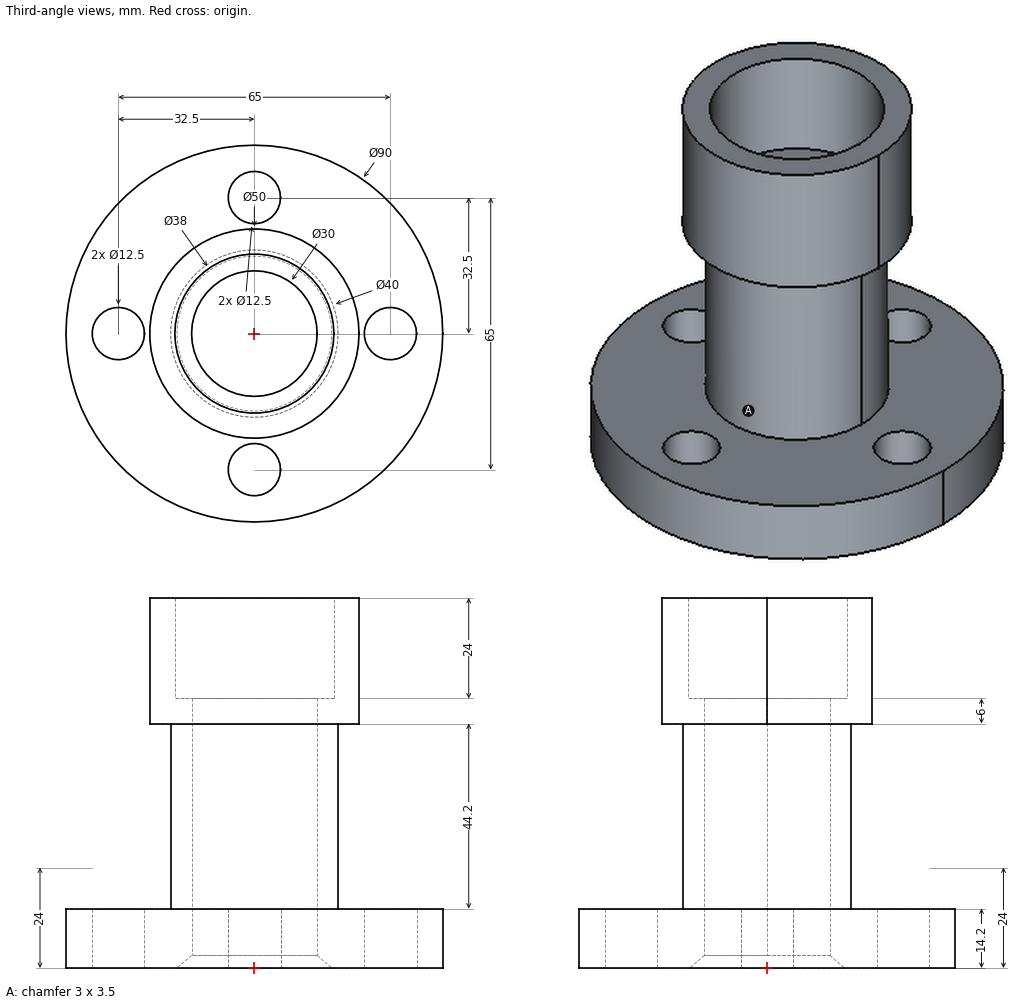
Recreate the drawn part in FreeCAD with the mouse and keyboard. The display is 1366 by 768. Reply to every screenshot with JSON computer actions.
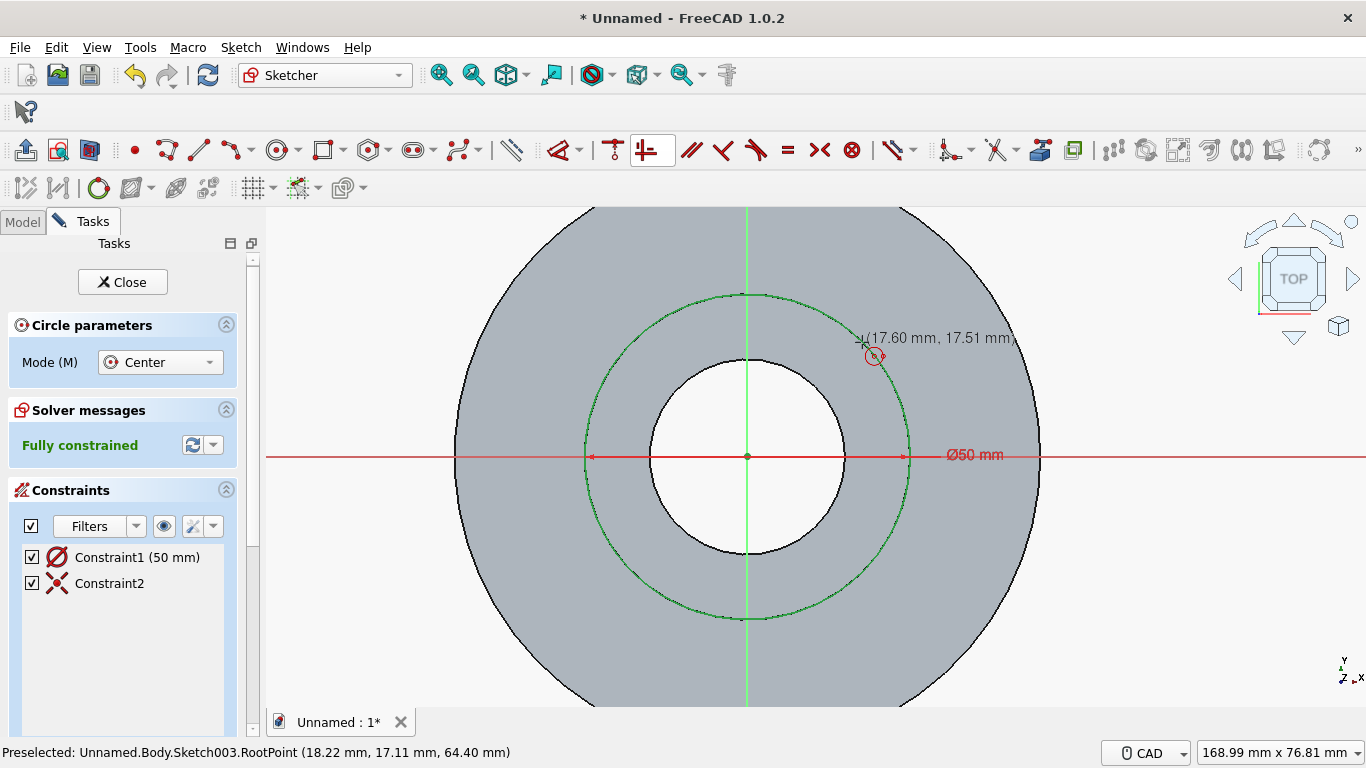
{"action": "left_click", "coordinate": [747, 457]}
{"action": "mouse_move", "coordinate": [835, 370]}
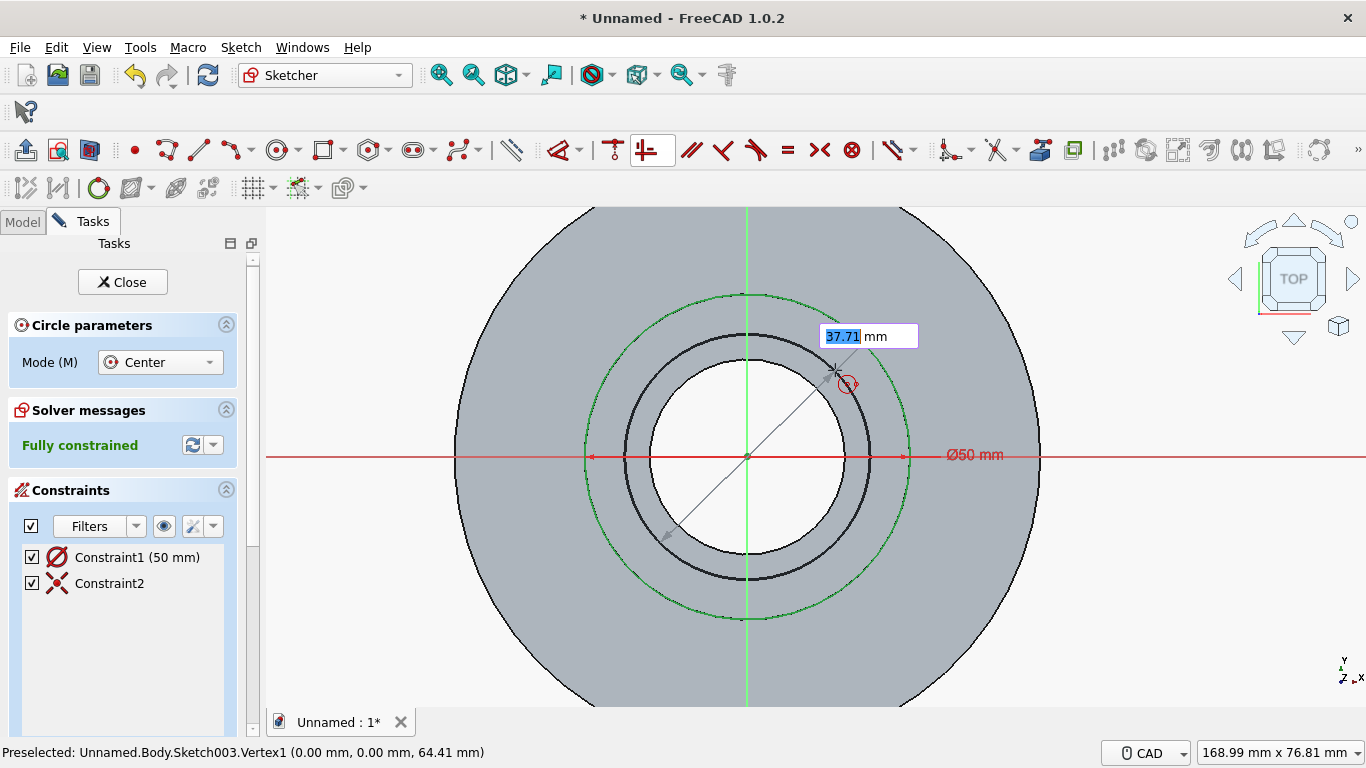
{"action": "type", "text": "38"}
{"action": "key", "text": "Return"}
{"action": "key", "text": "Escape"}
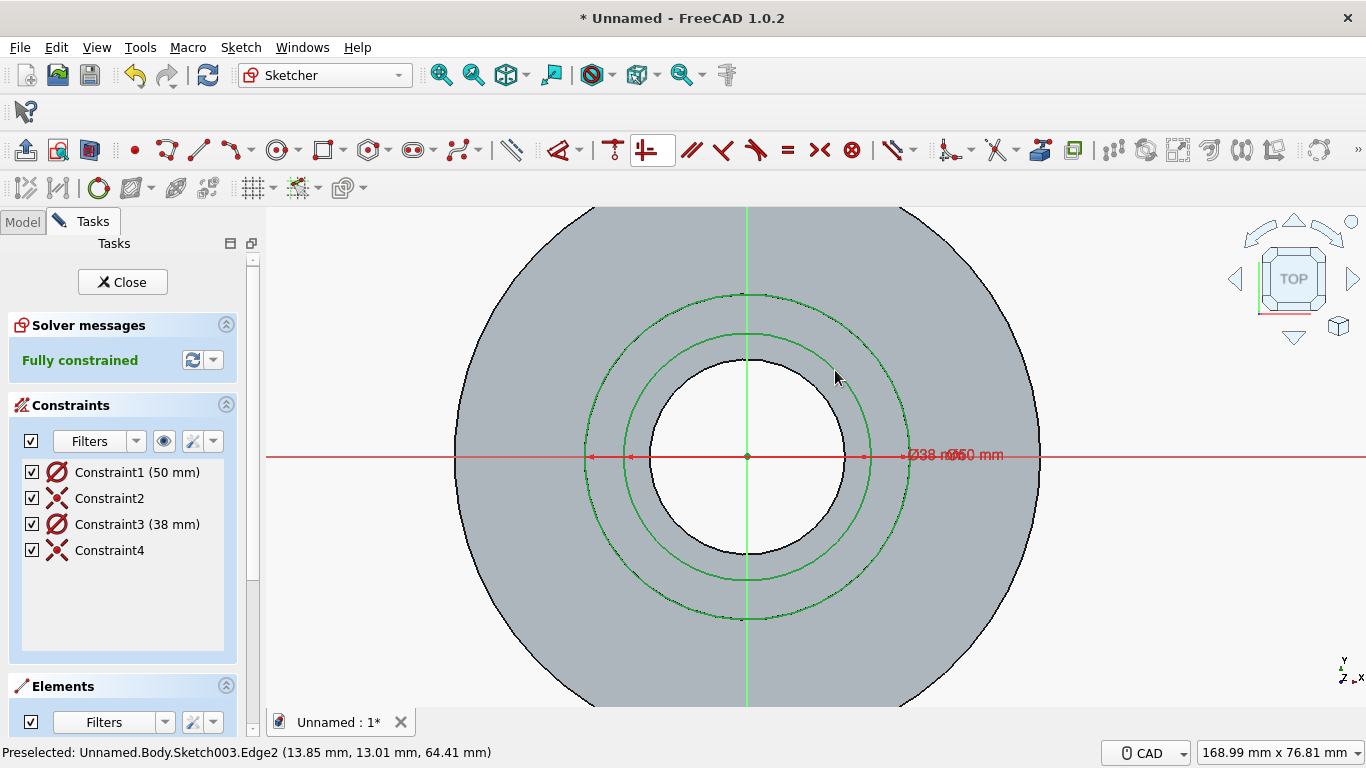
{"action": "left_click", "coordinate": [123, 282]}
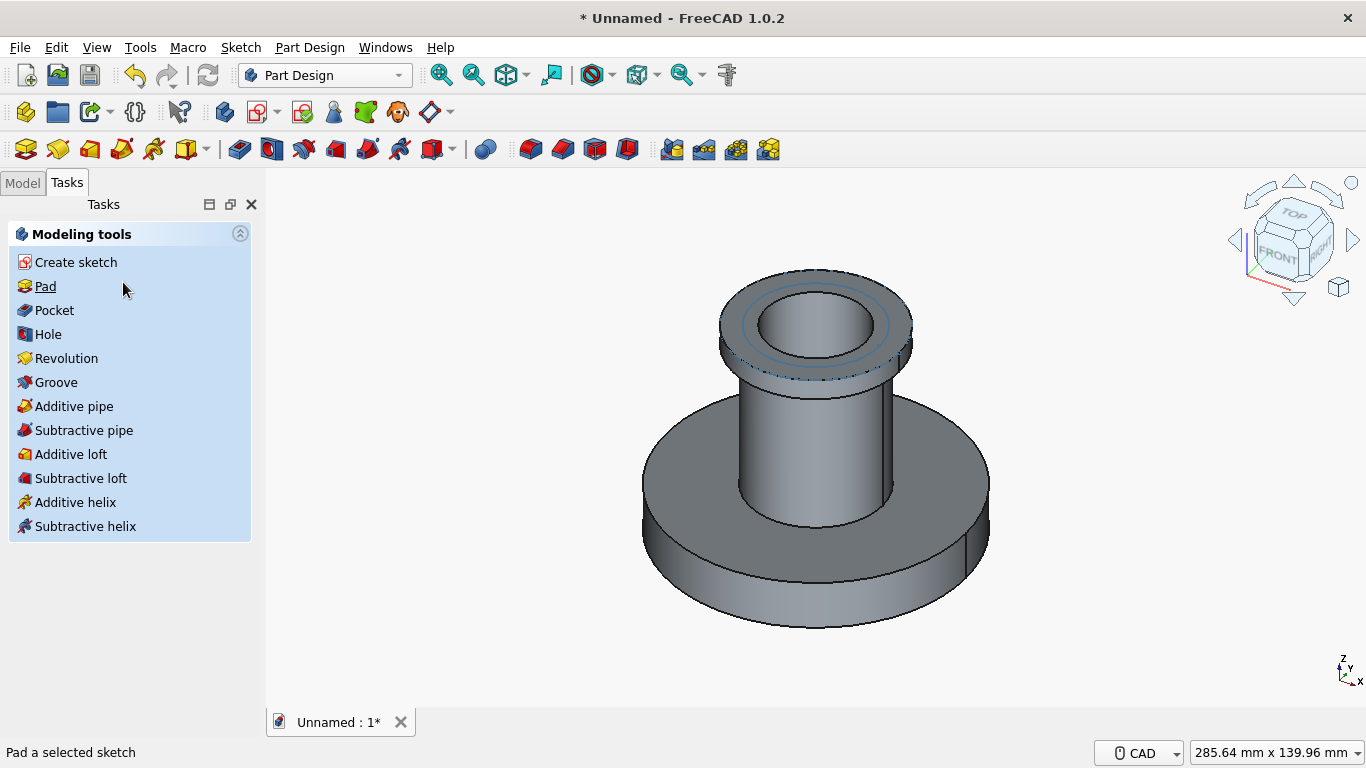
{"action": "left_click", "coordinate": [26, 150]}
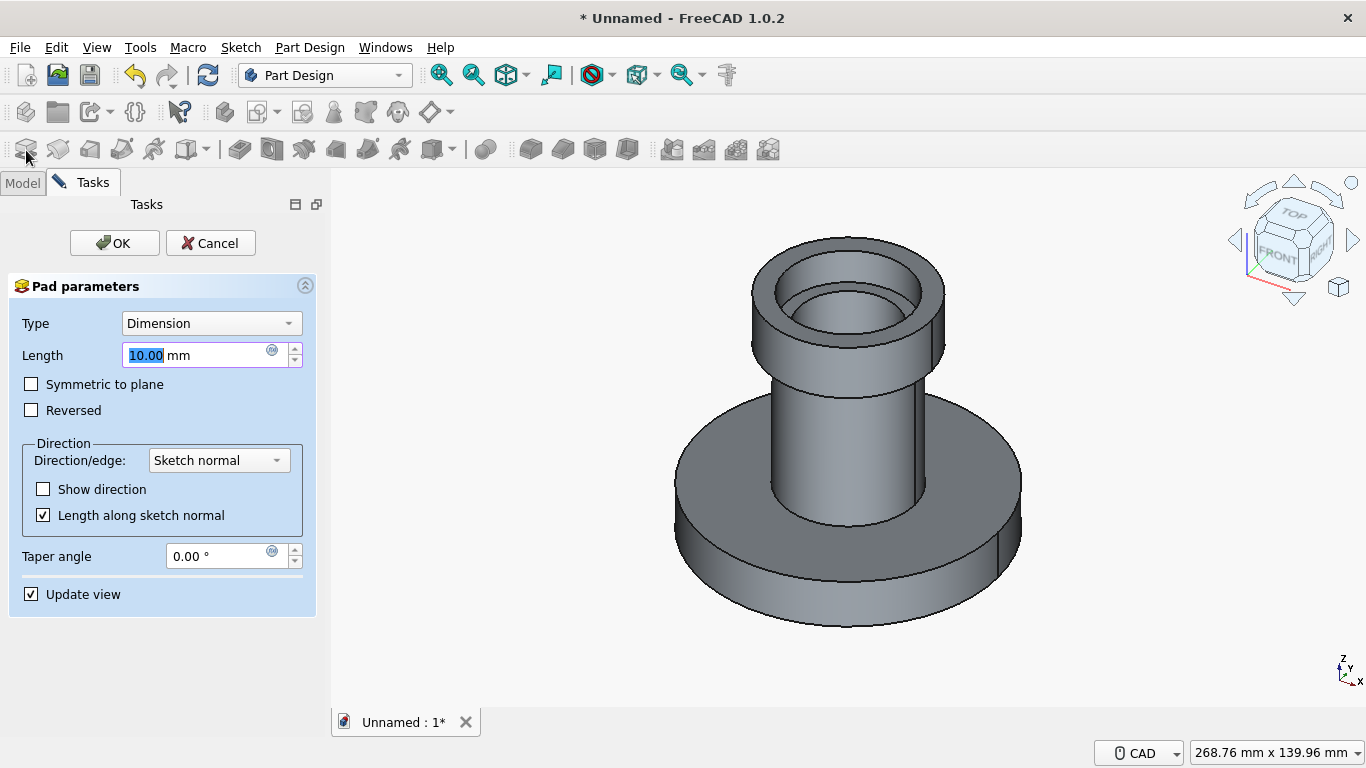
{"action": "type", "text": "24"}
{"action": "key", "text": "Tab"}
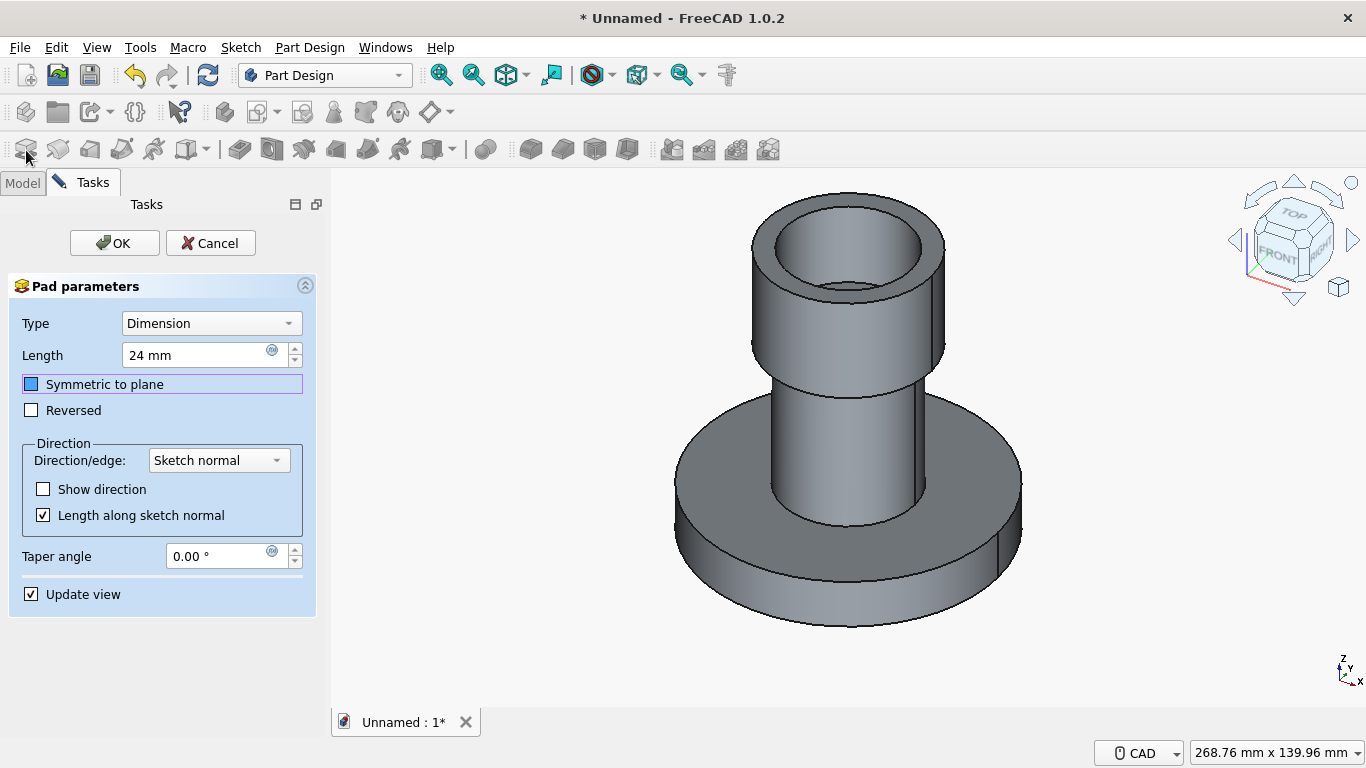
{"action": "left_click", "coordinate": [115, 243]}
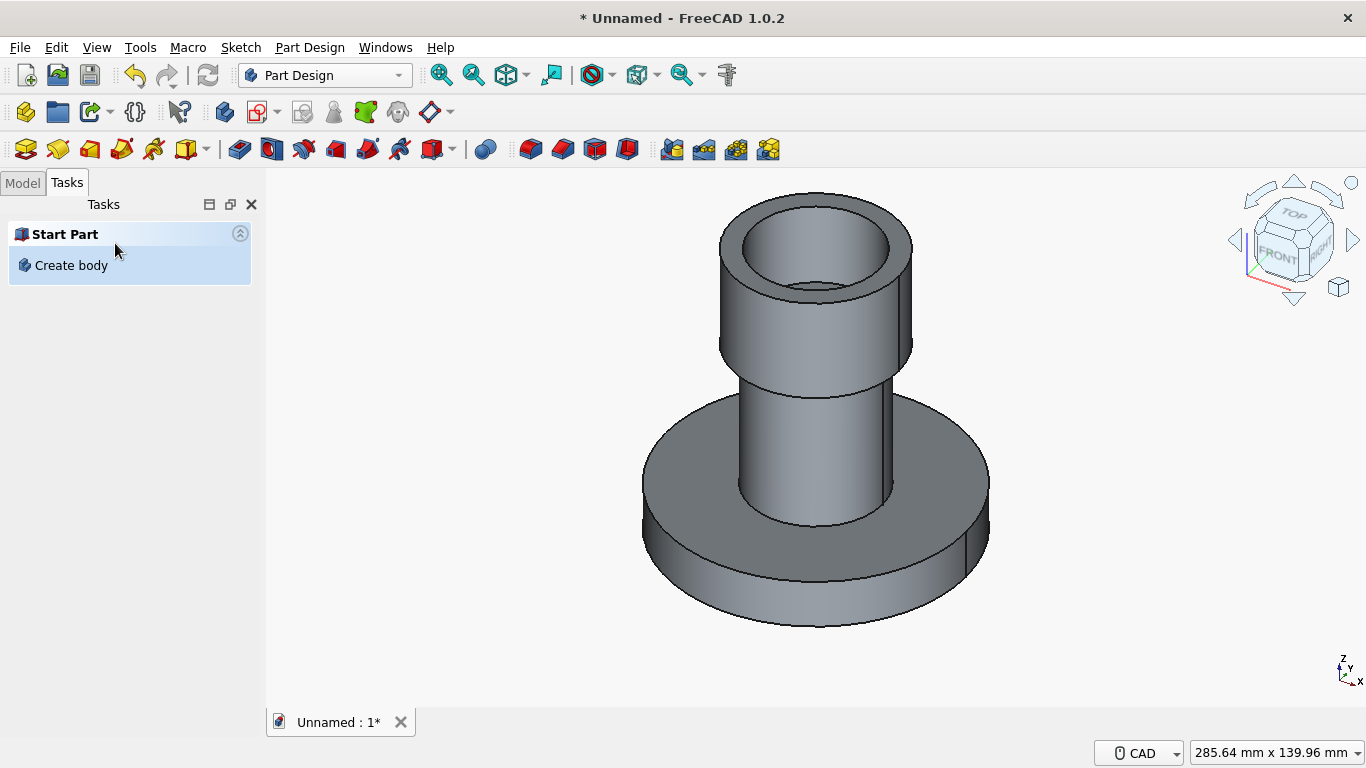
{"action": "key", "text": "v f"}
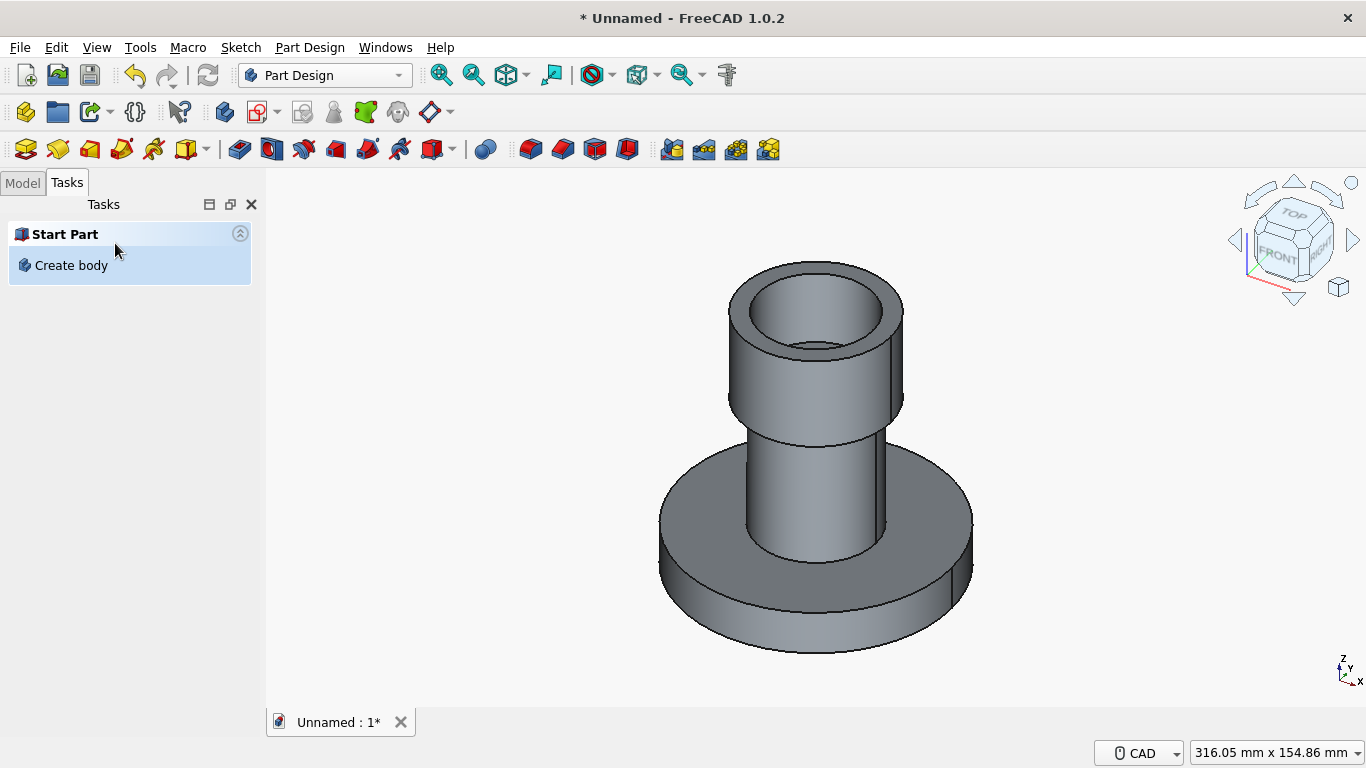
{"action": "key", "text": "0"}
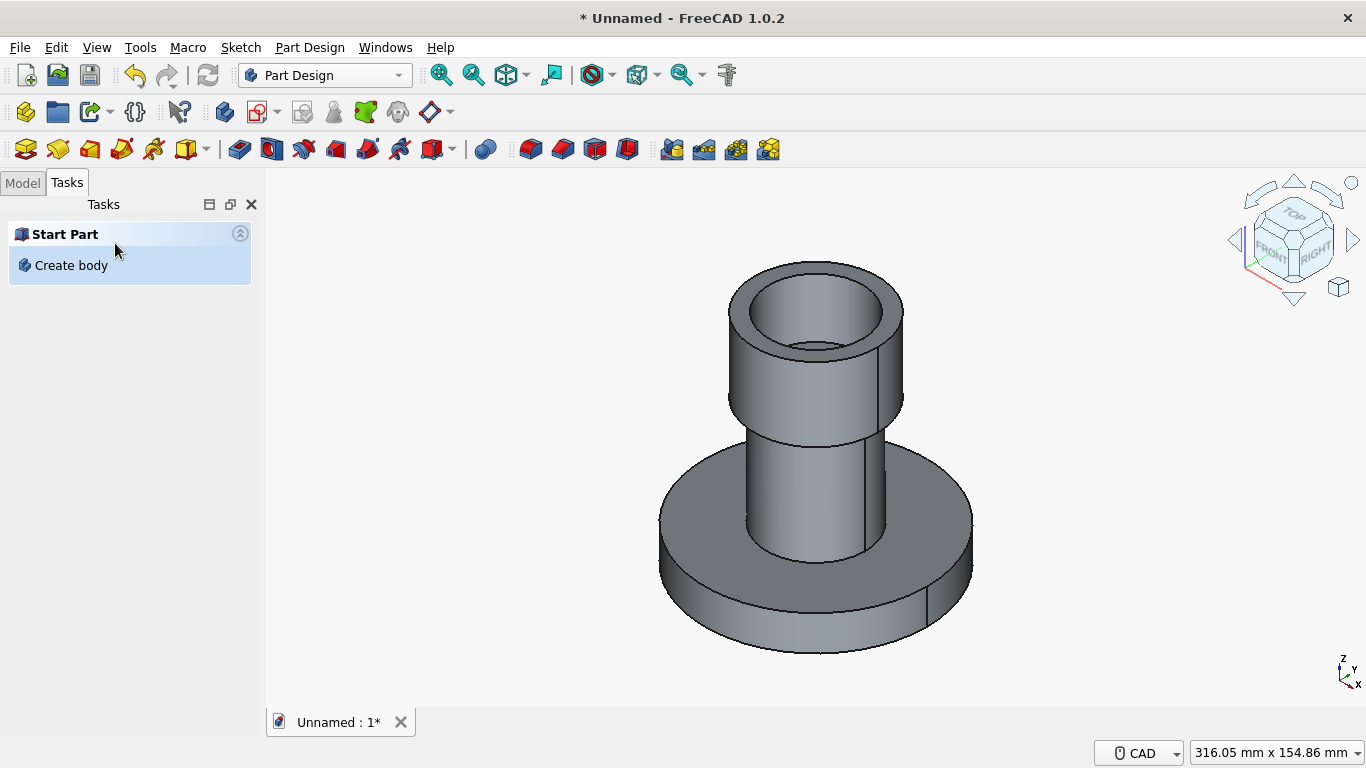
{"action": "key", "text": "2"}